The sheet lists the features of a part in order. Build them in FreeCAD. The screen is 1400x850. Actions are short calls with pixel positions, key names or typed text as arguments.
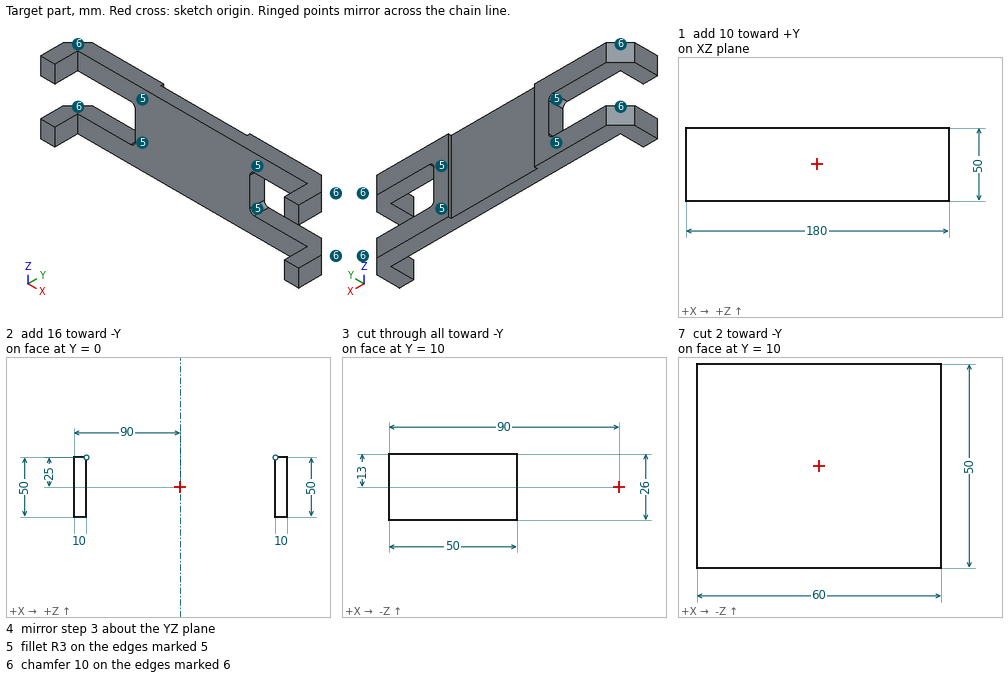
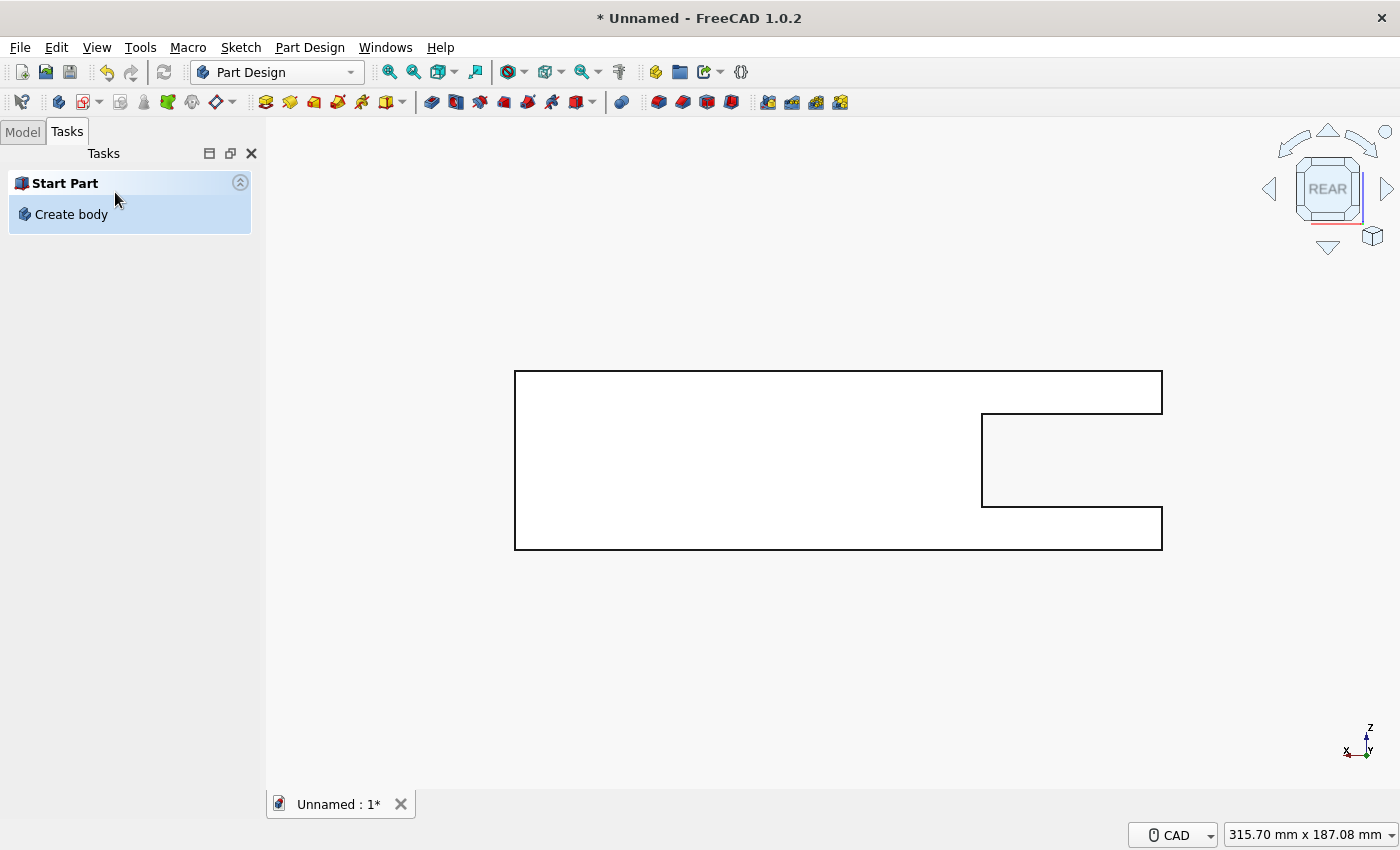
click(23, 131)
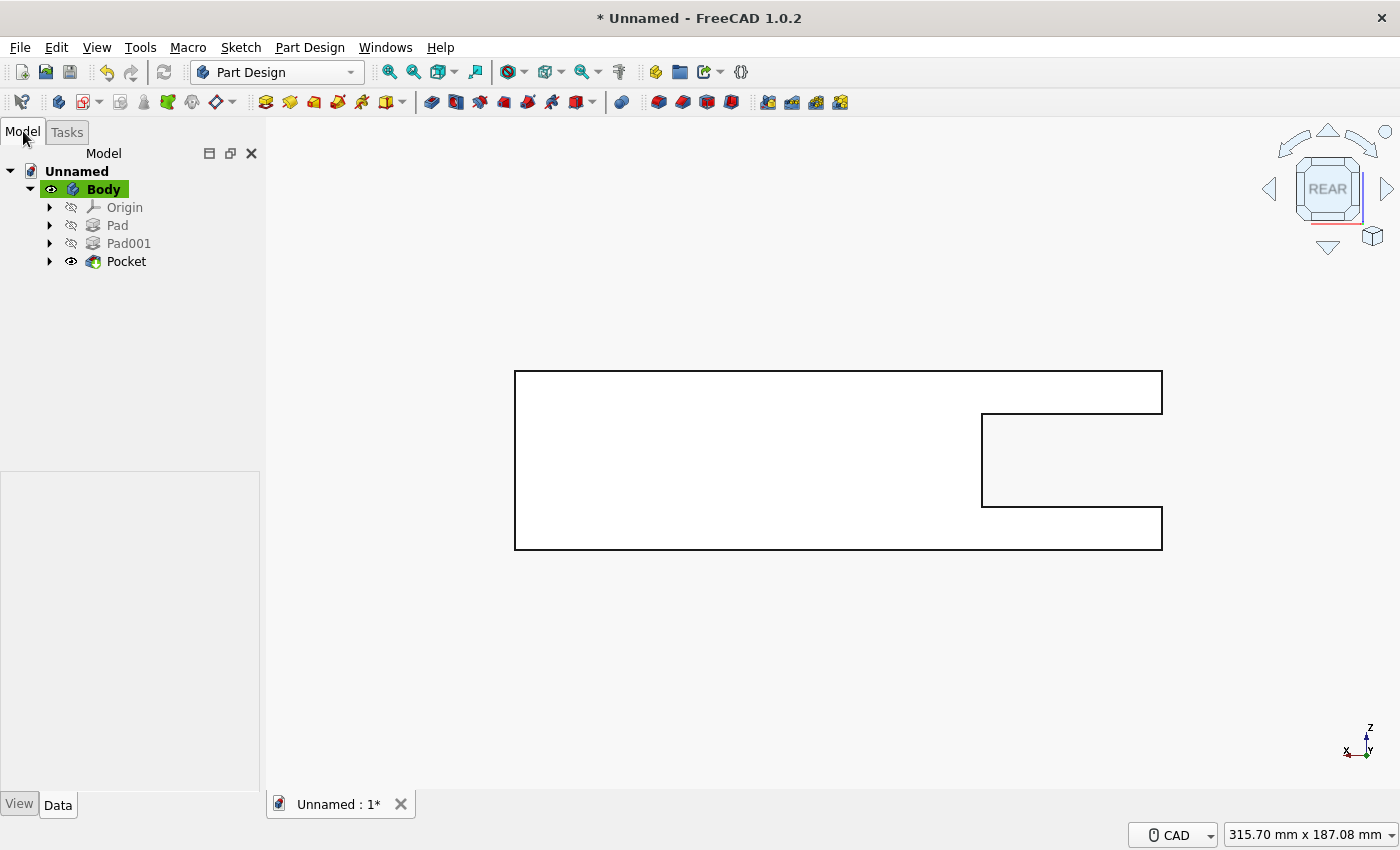
click(116, 261)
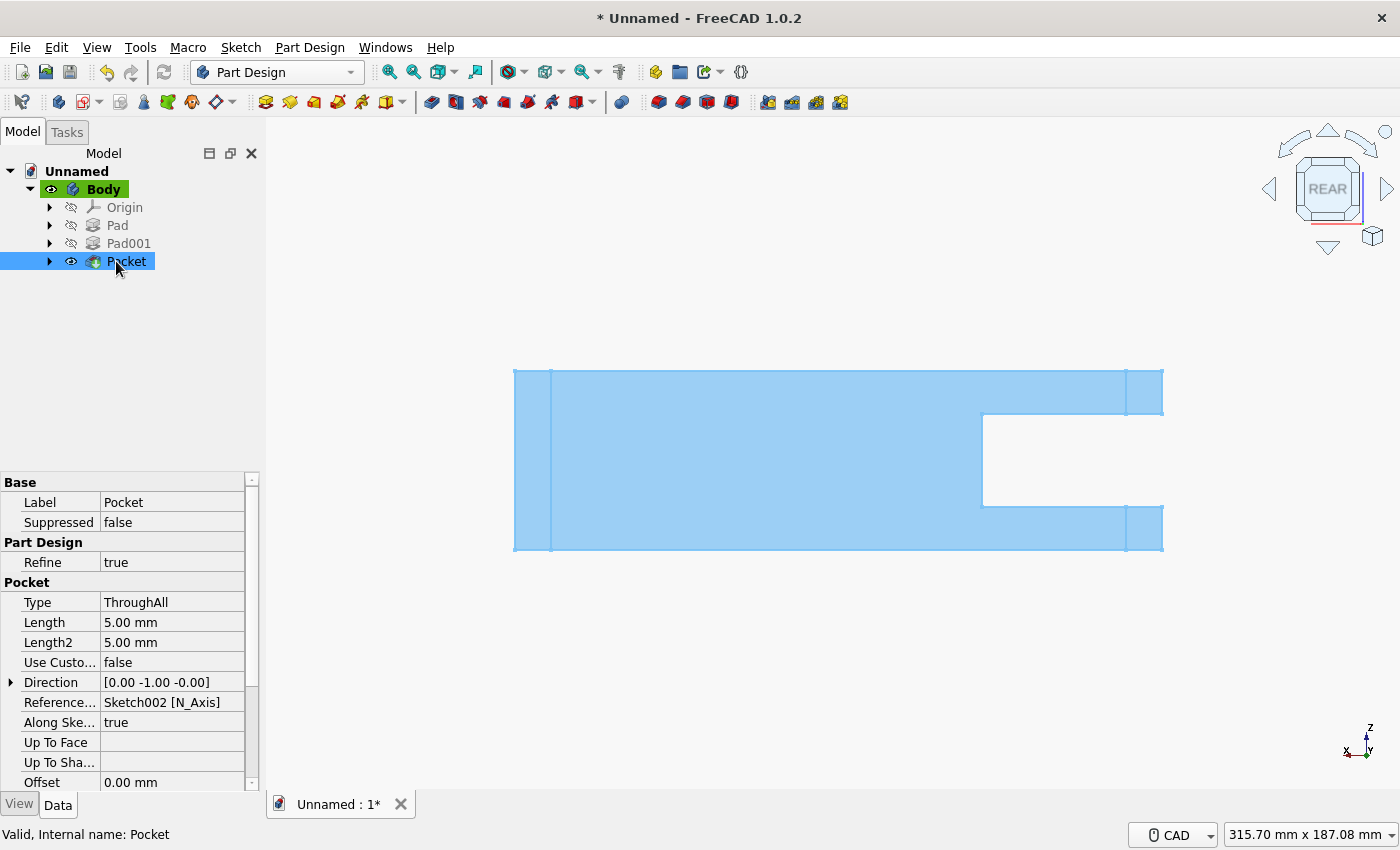
click(768, 102)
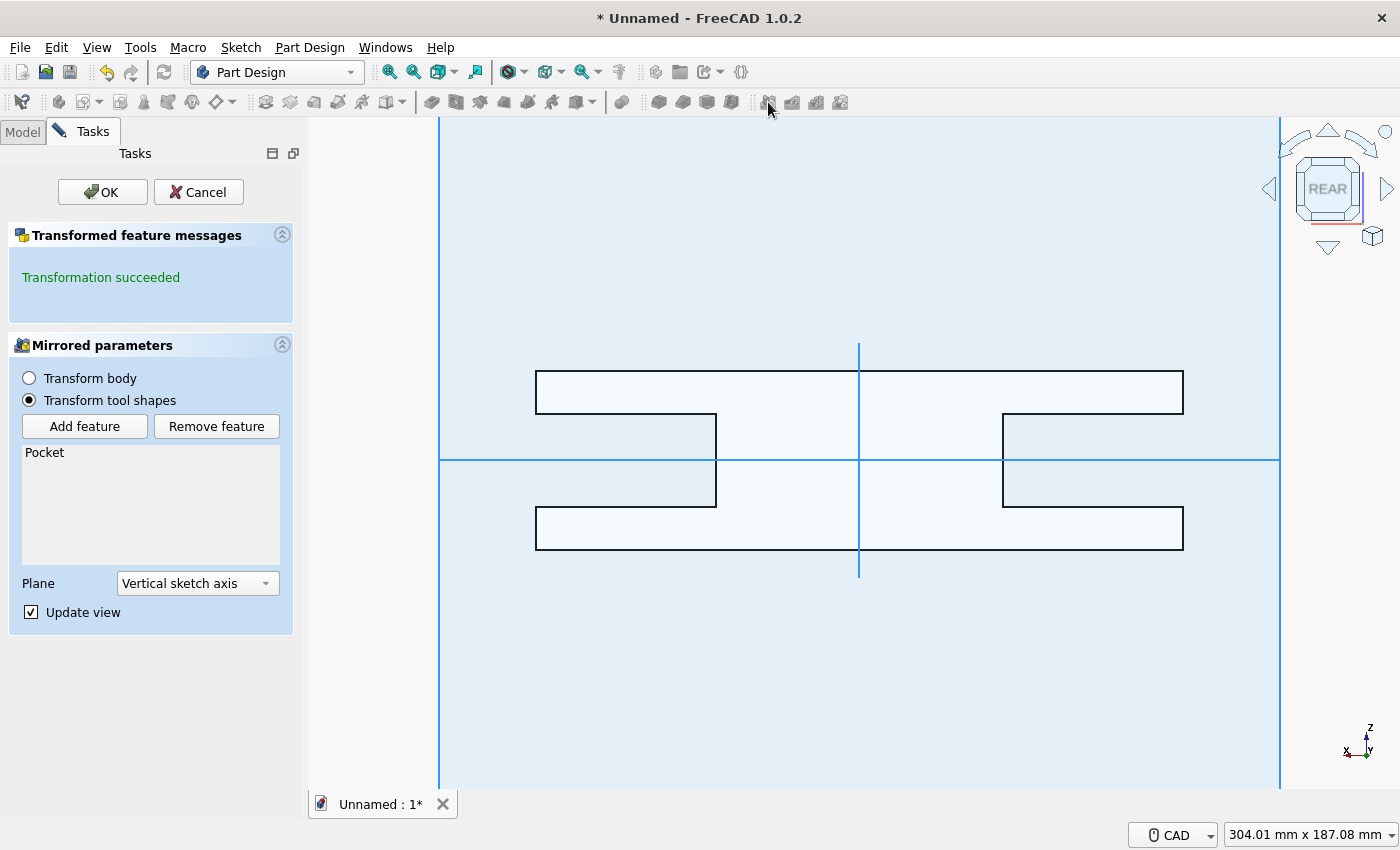
click(198, 584)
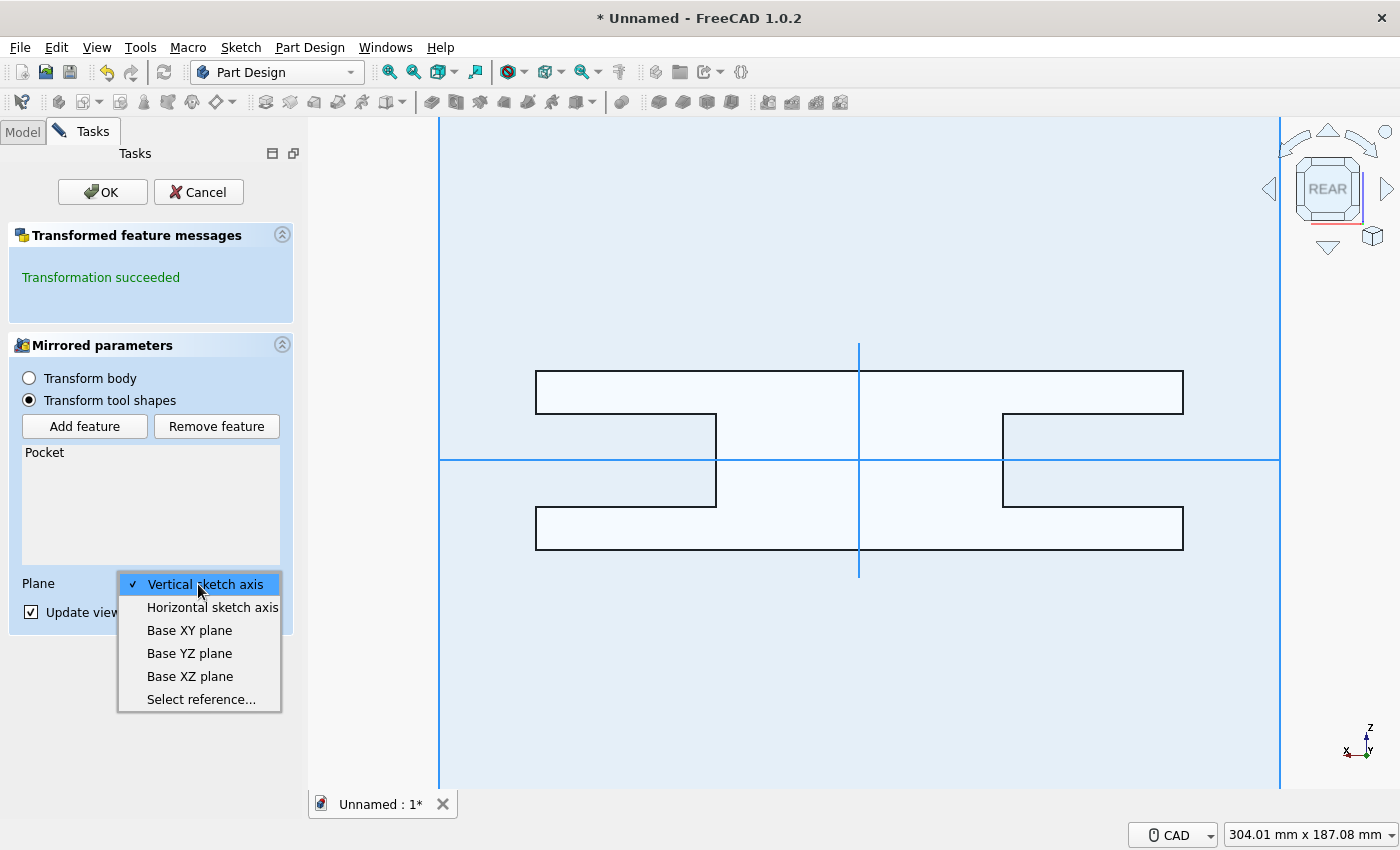
click(198, 654)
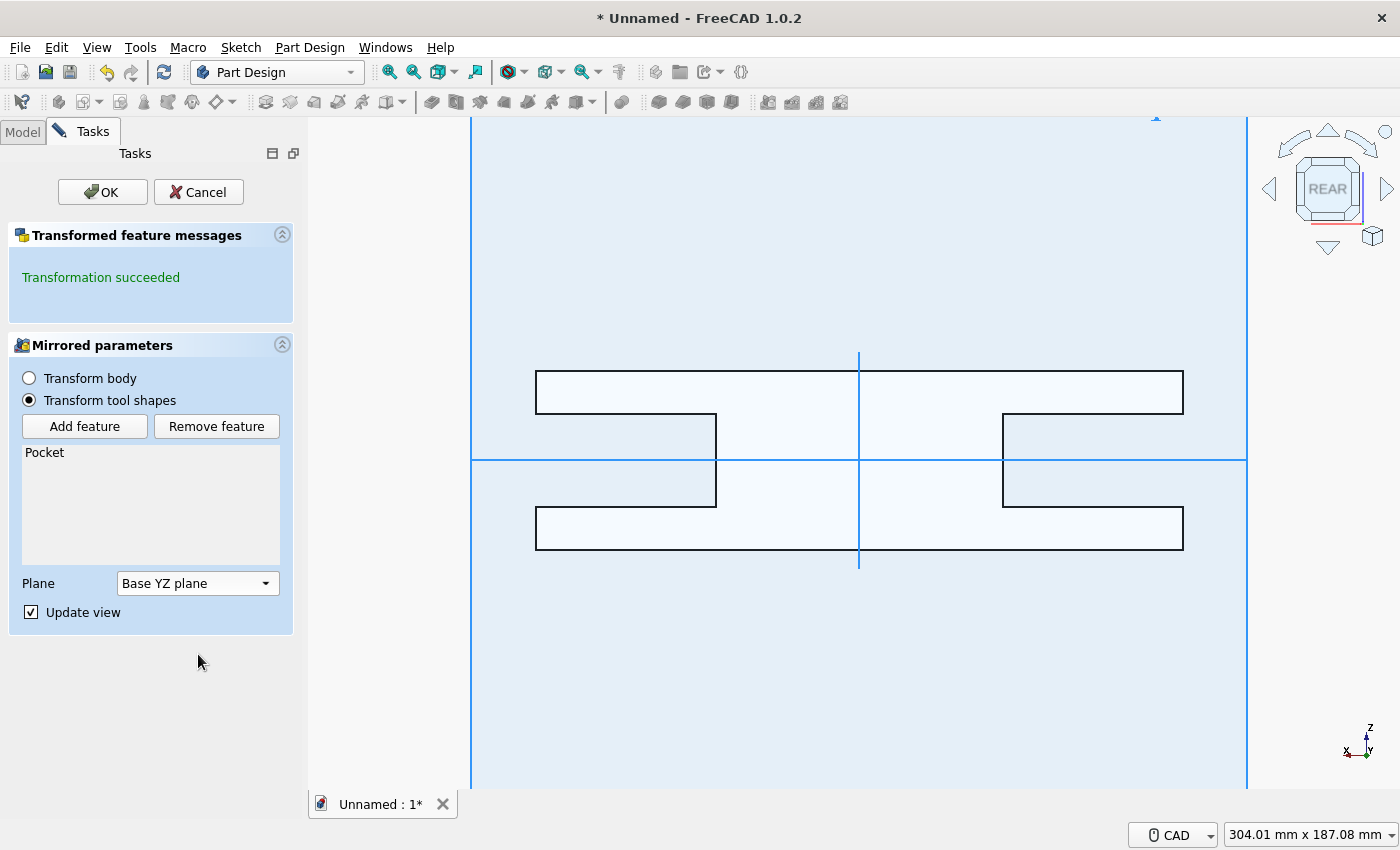
click(103, 192)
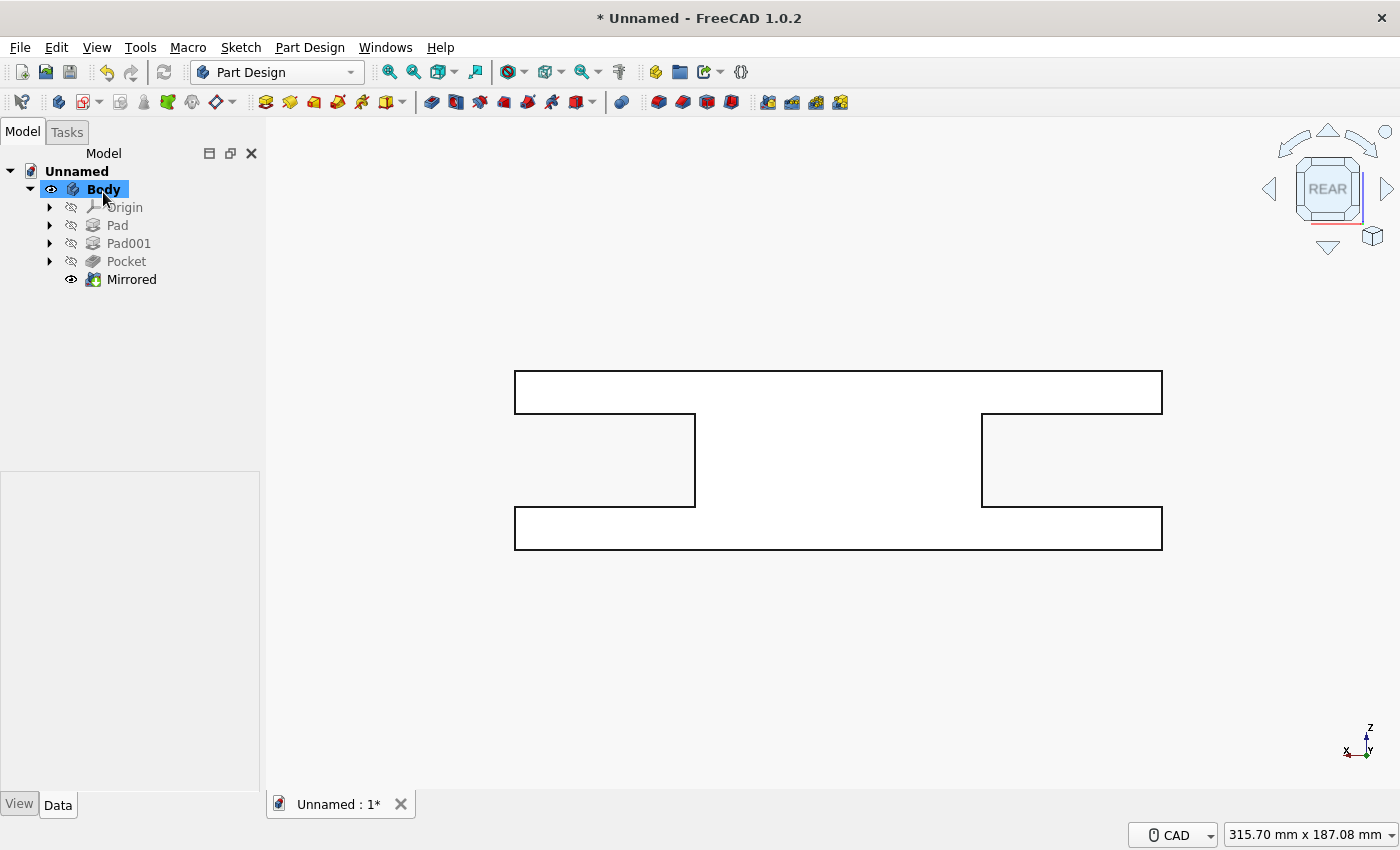
key(0)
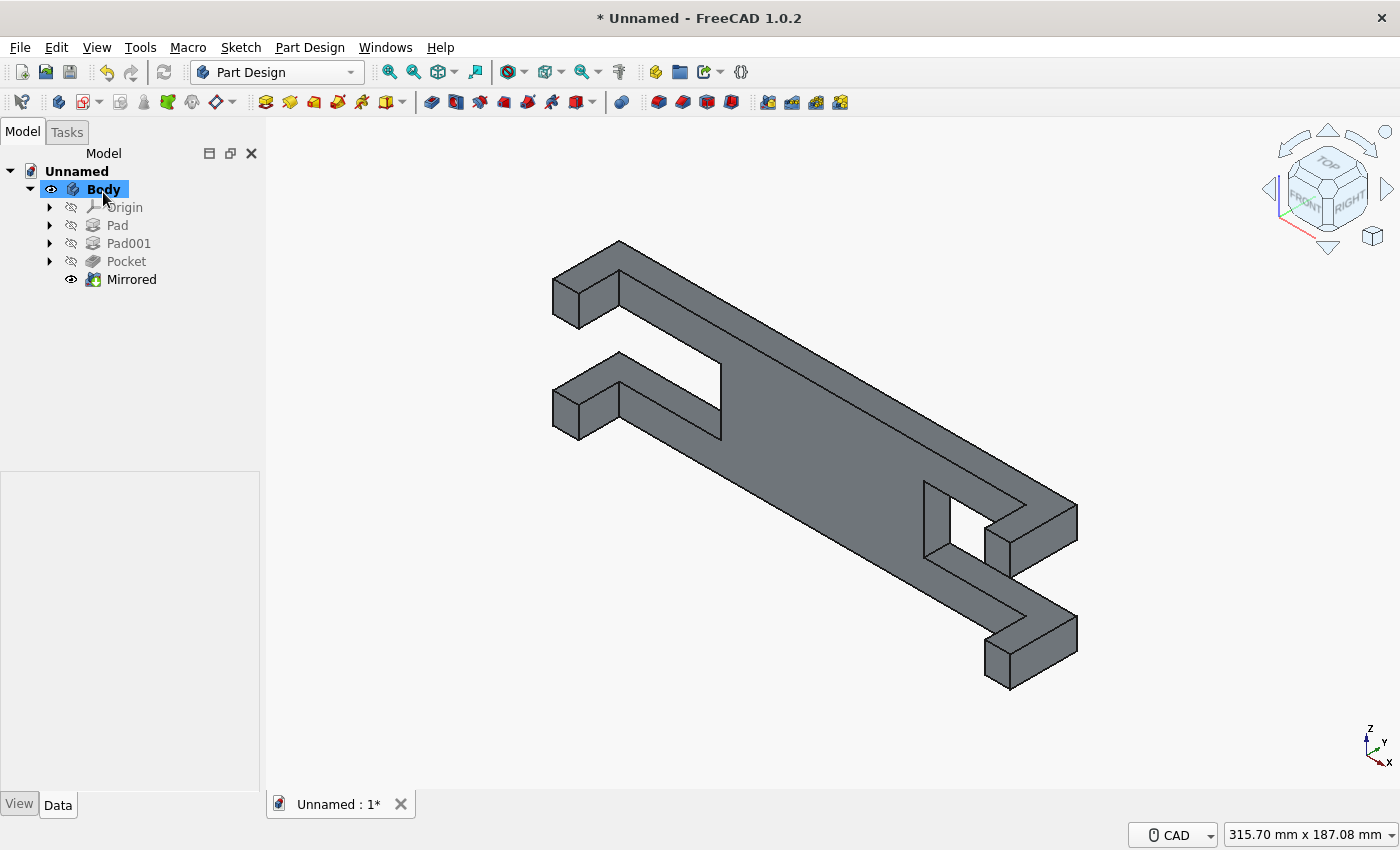
key(2)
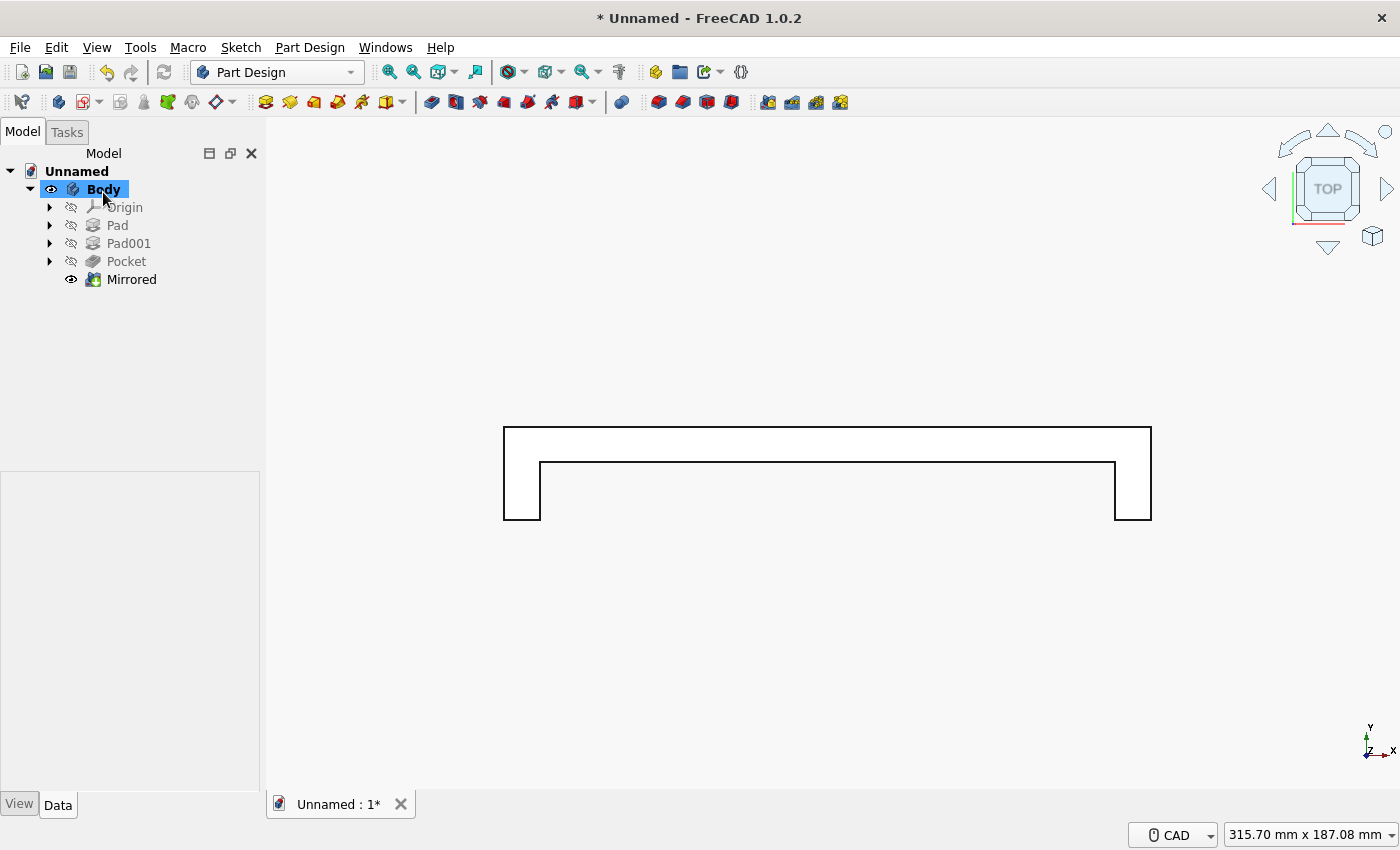
key(1)